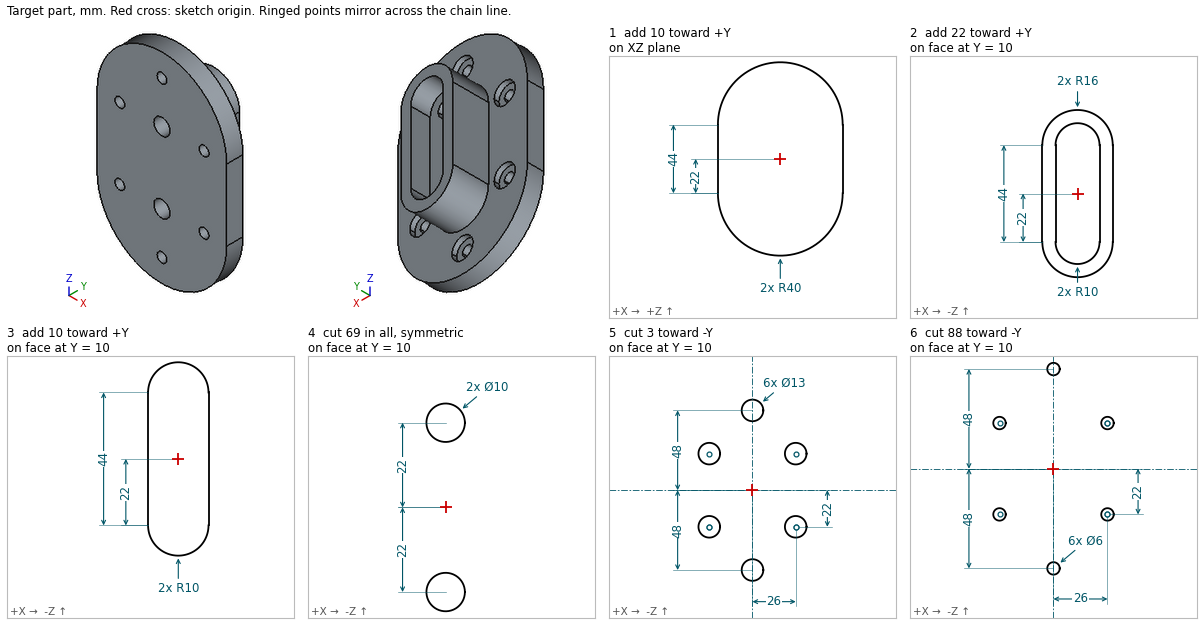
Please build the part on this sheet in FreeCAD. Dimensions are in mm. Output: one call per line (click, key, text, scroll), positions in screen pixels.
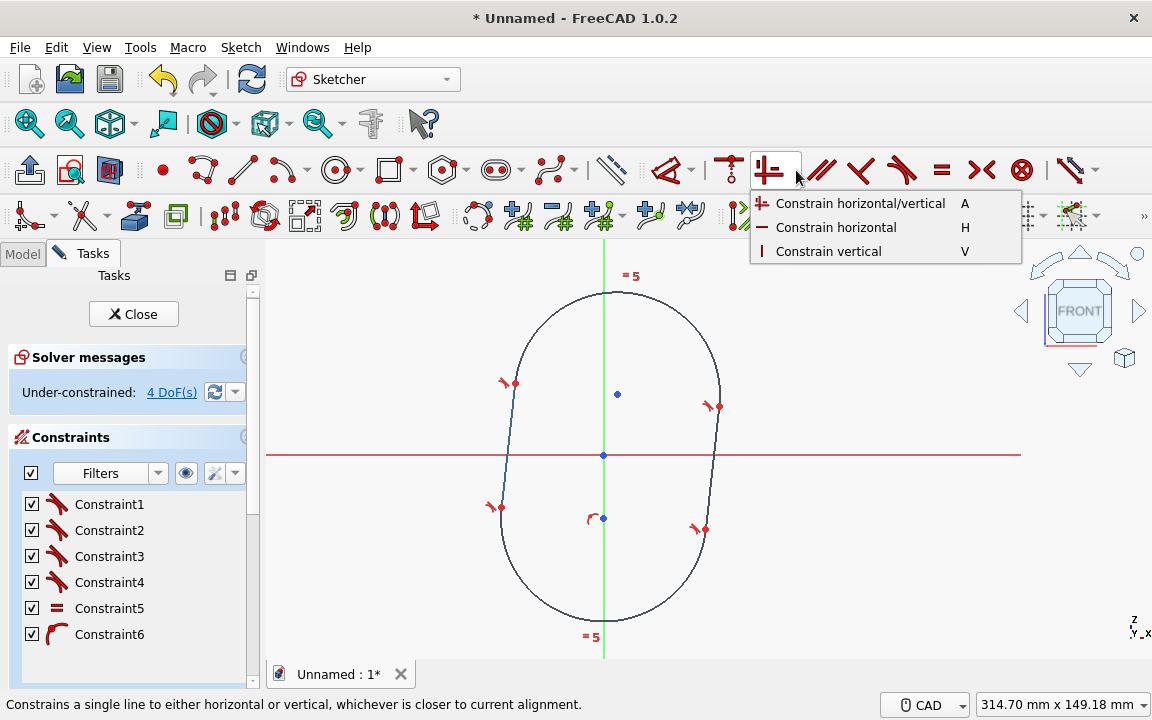
click(886, 251)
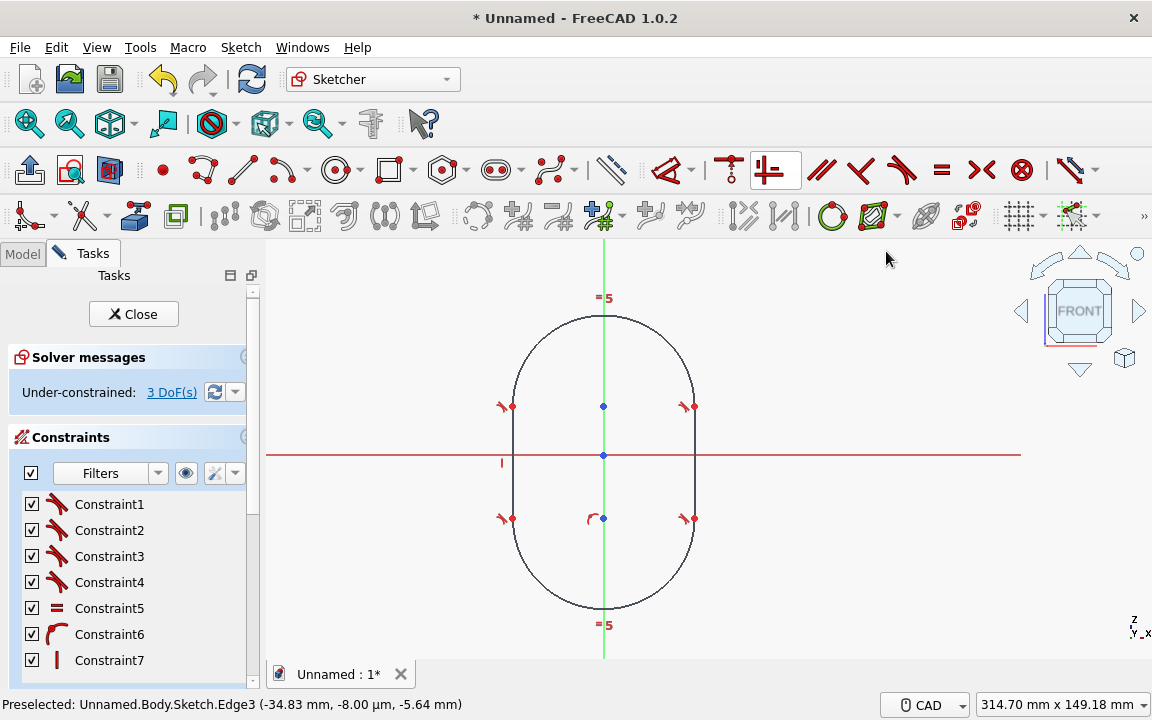
click(666, 170)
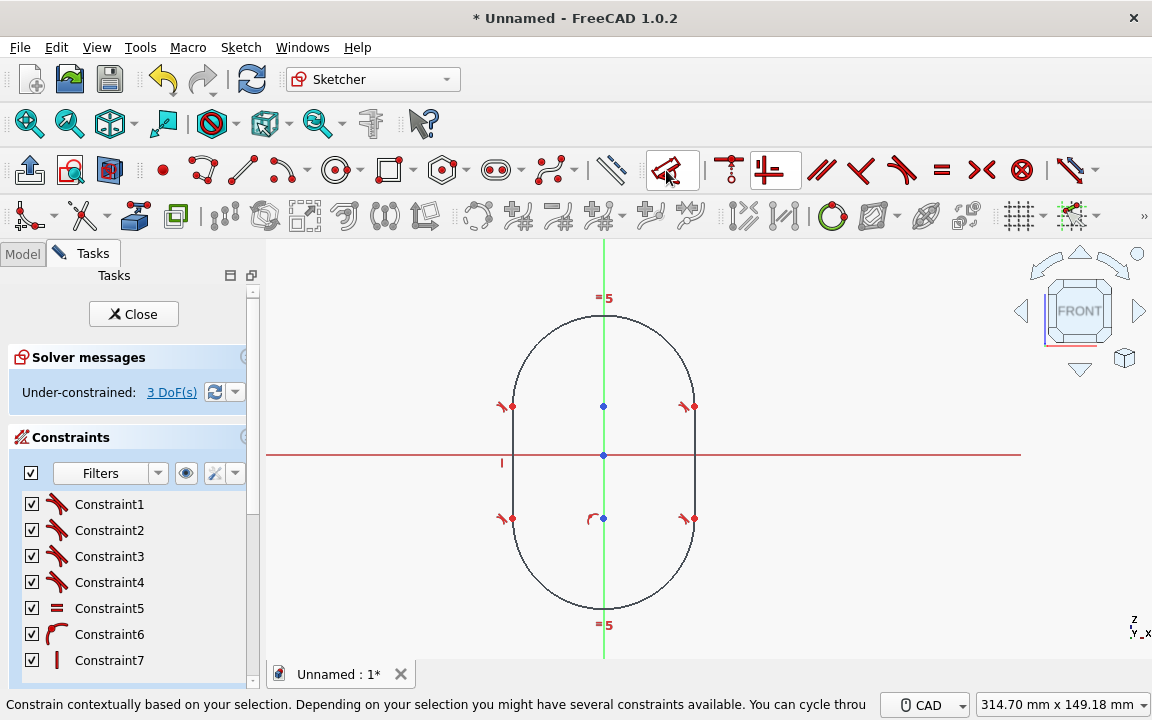
click(550, 592)
click(531, 618)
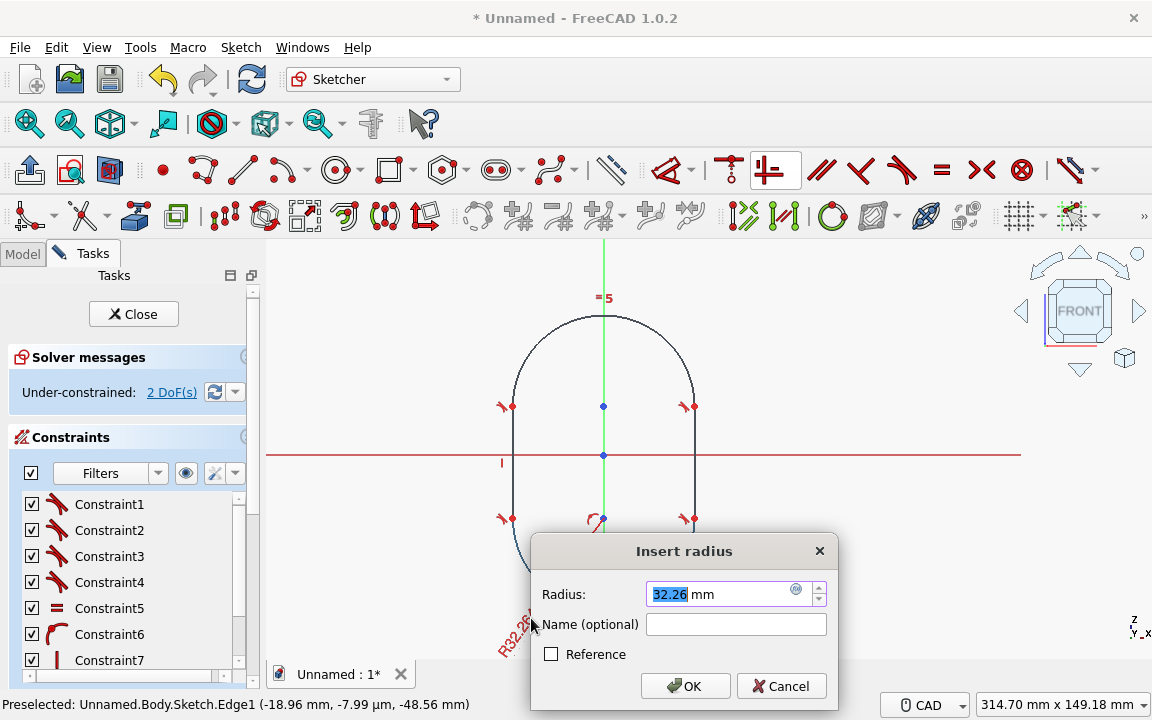
text(40)
key(Return)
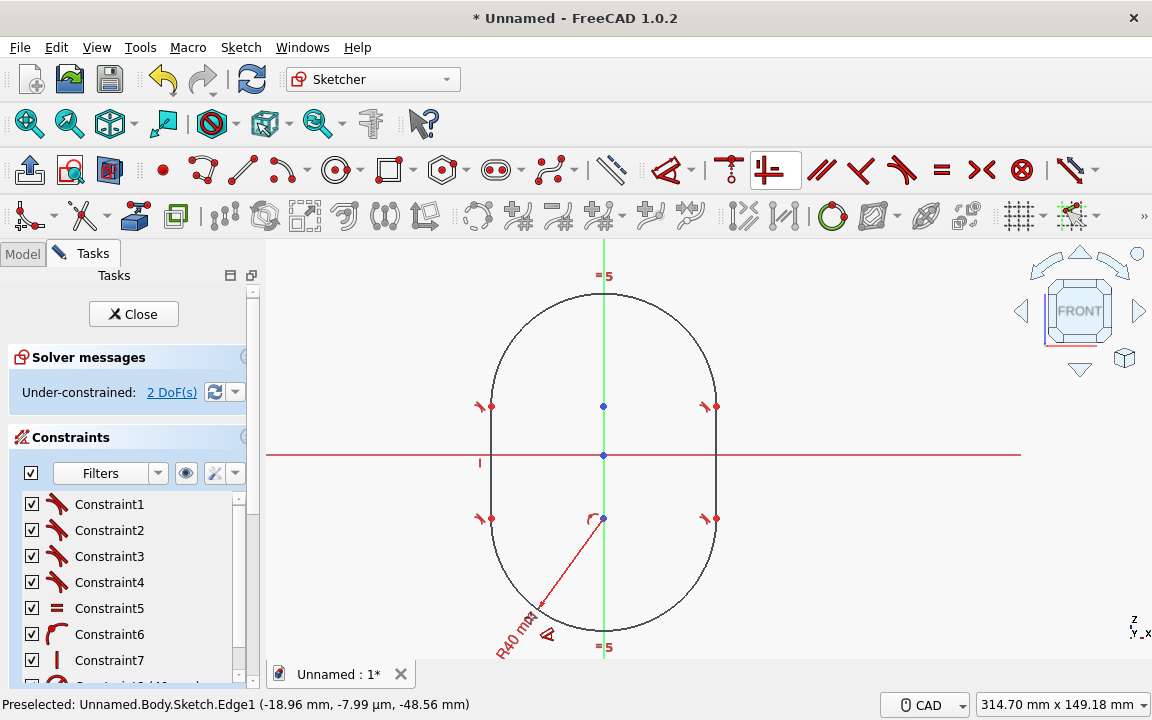
click(491, 485)
click(457, 437)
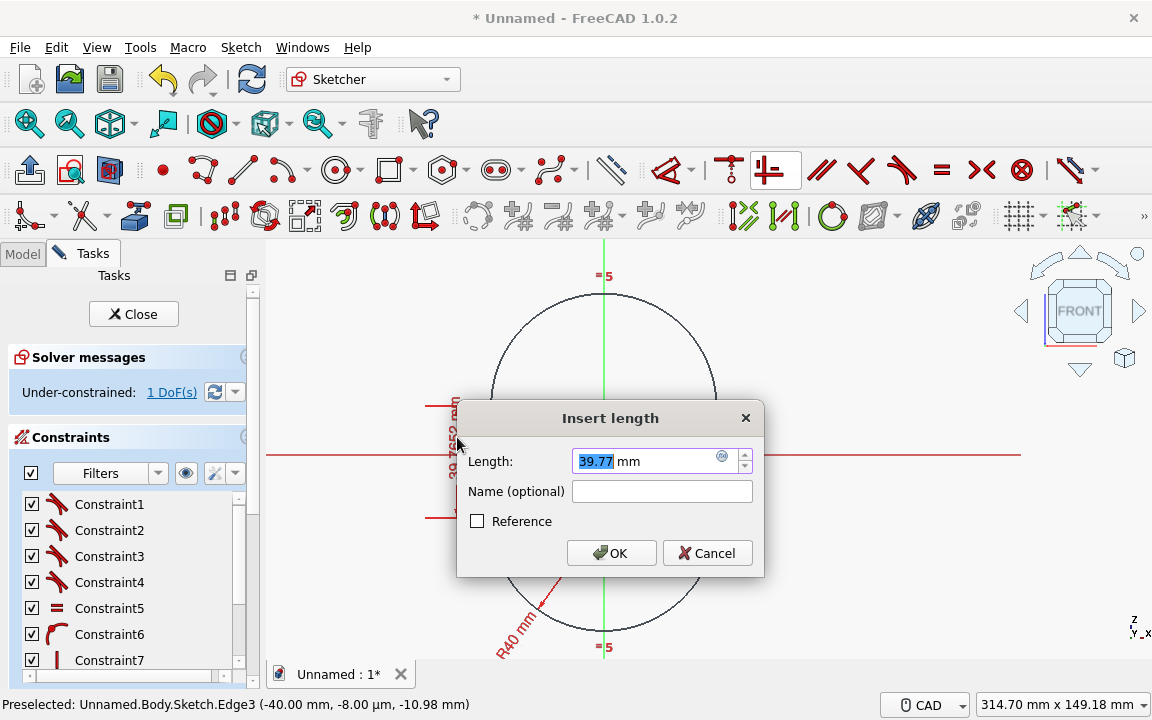
text(44)
key(Return)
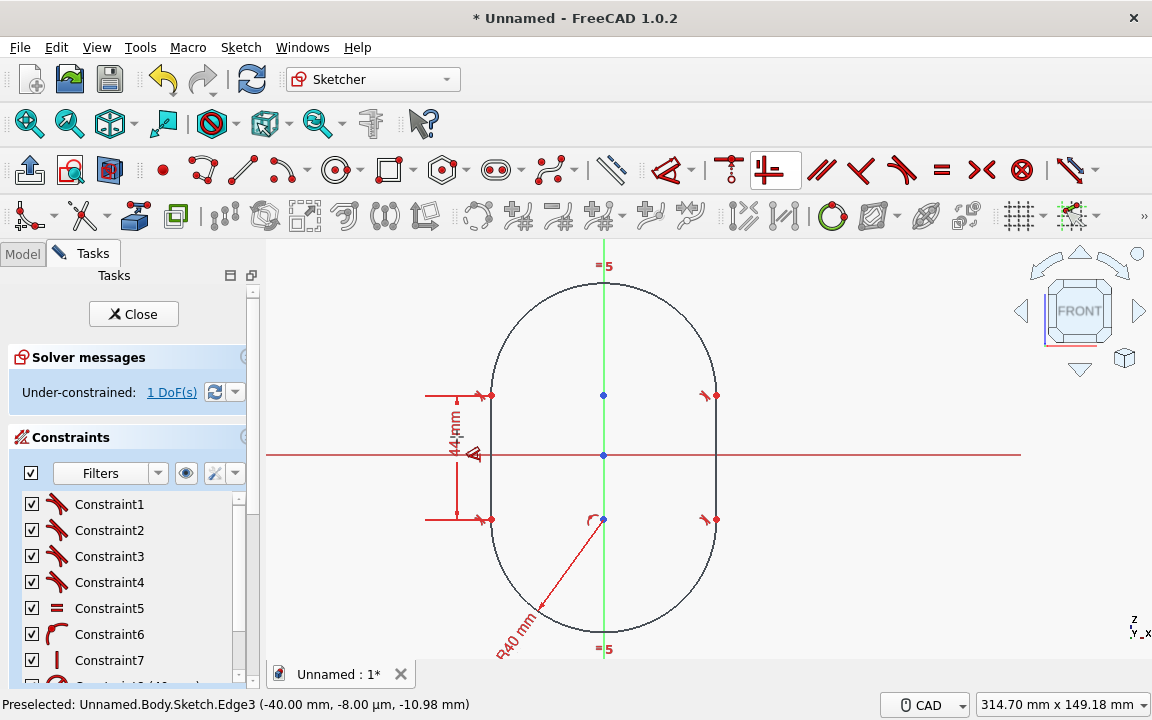
click(491, 520)
click(457, 487)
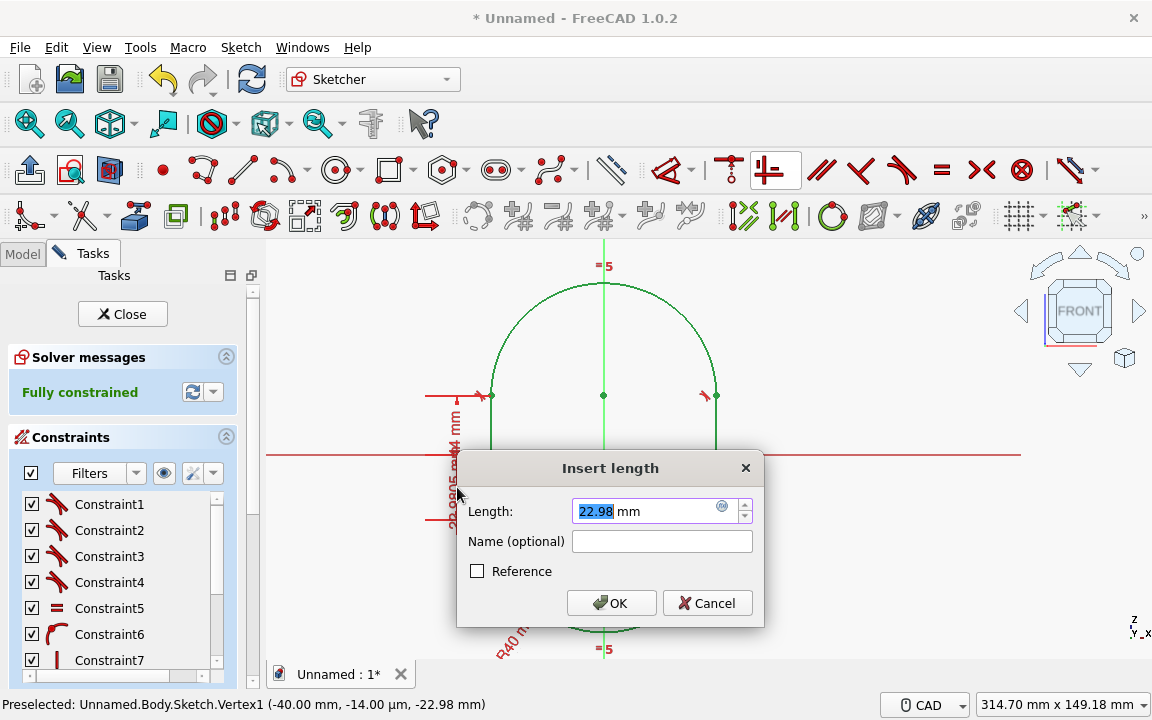
text(22)
key(Return)
key(Escape)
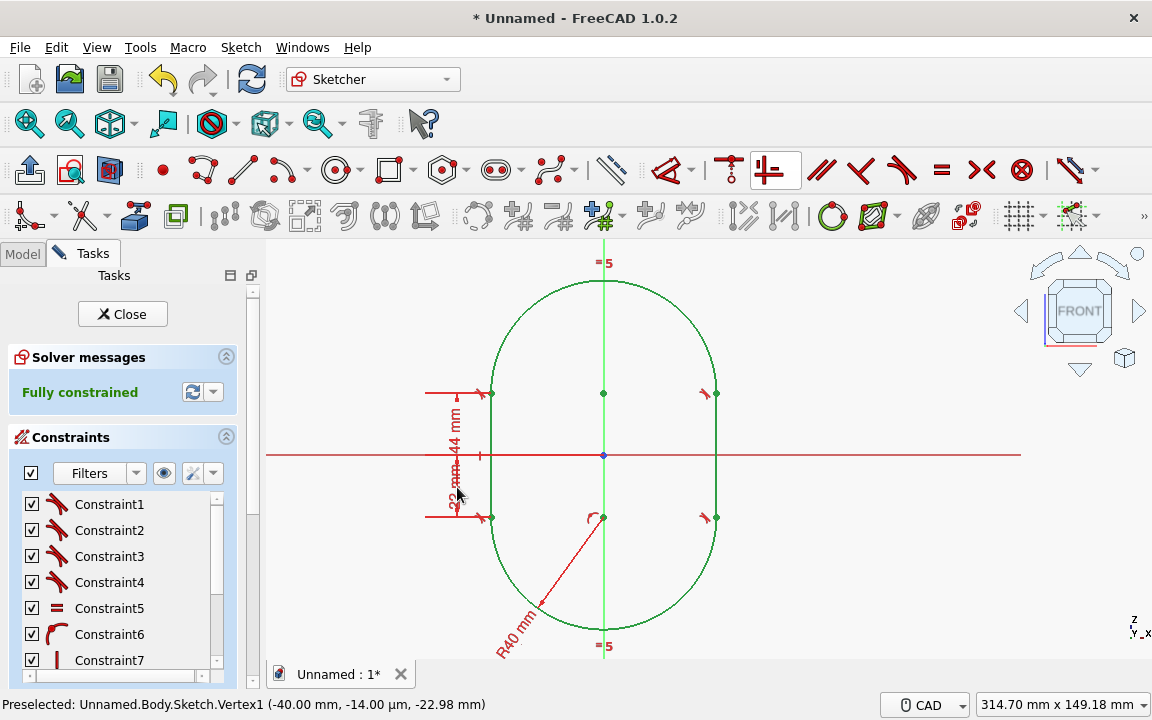
click(123, 314)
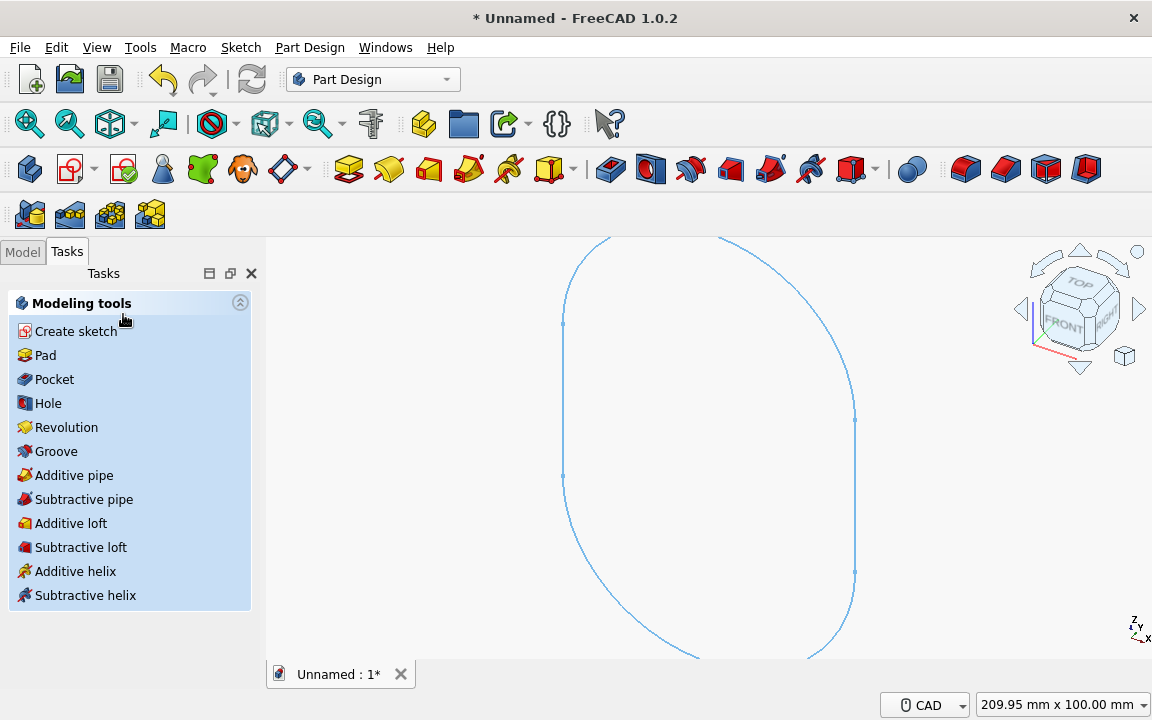
click(350, 170)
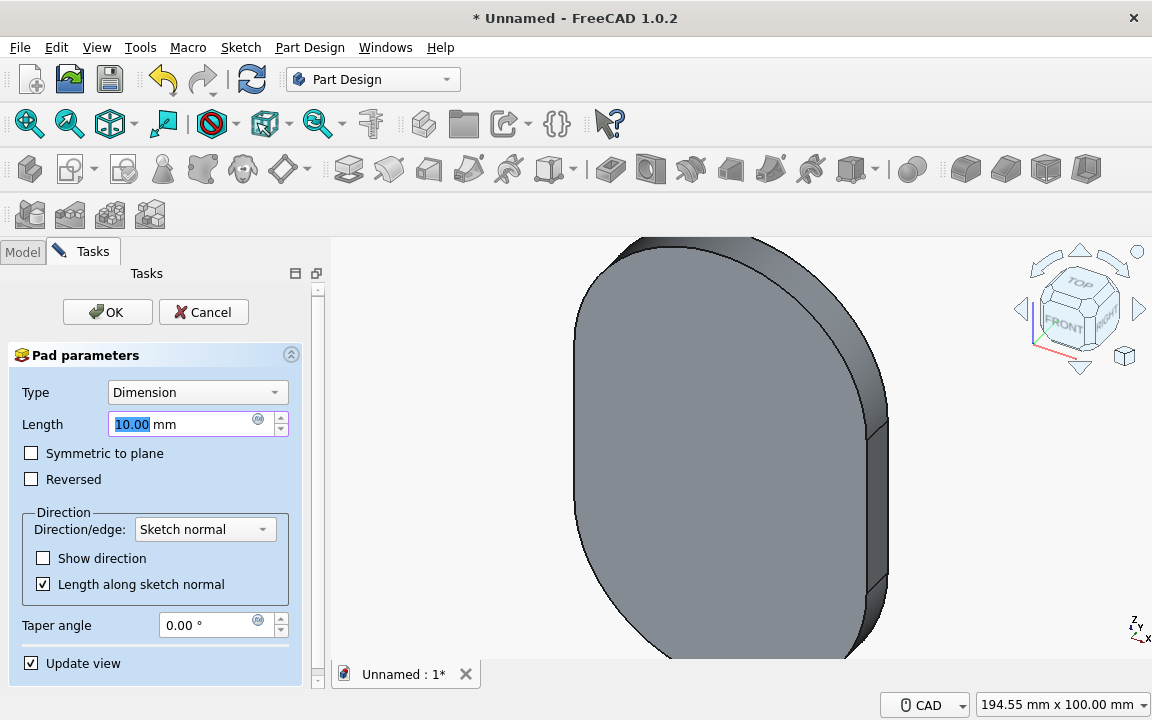
text(10)
key(Tab)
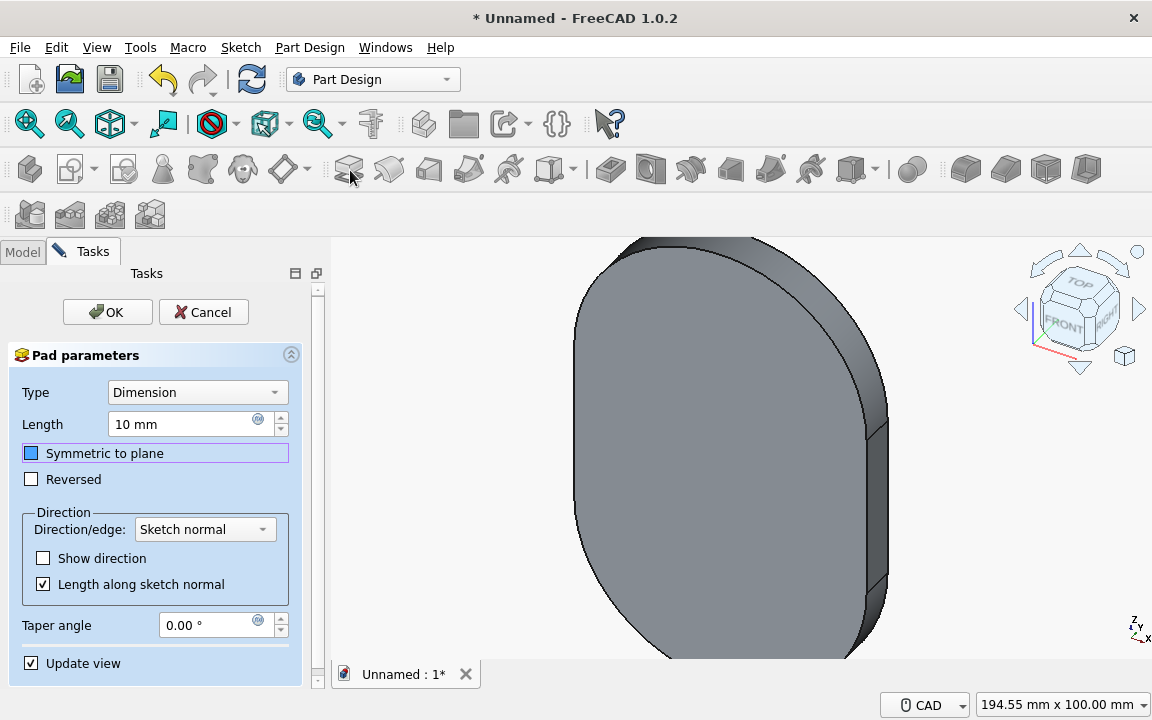
click(30, 479)